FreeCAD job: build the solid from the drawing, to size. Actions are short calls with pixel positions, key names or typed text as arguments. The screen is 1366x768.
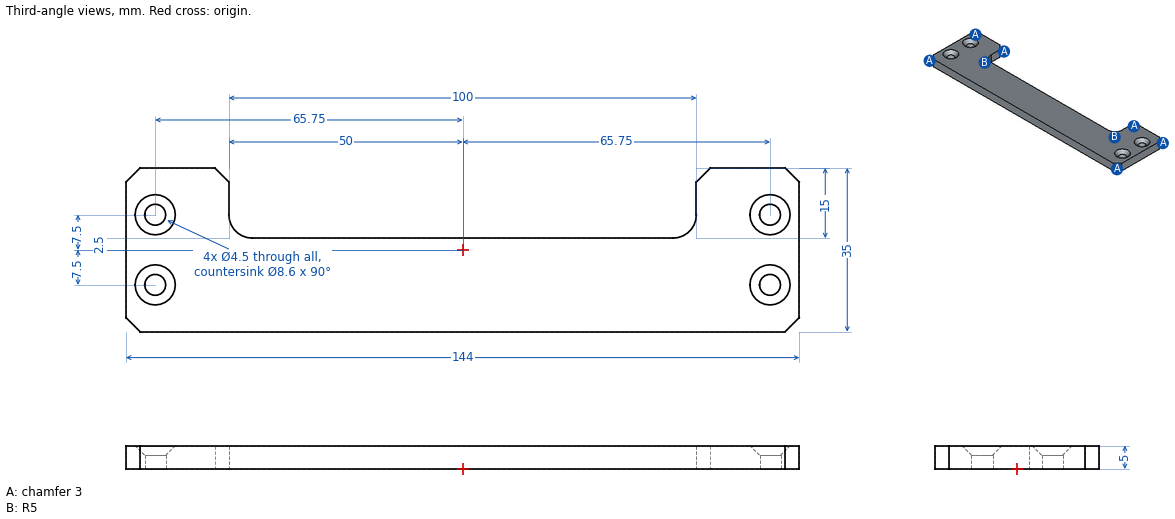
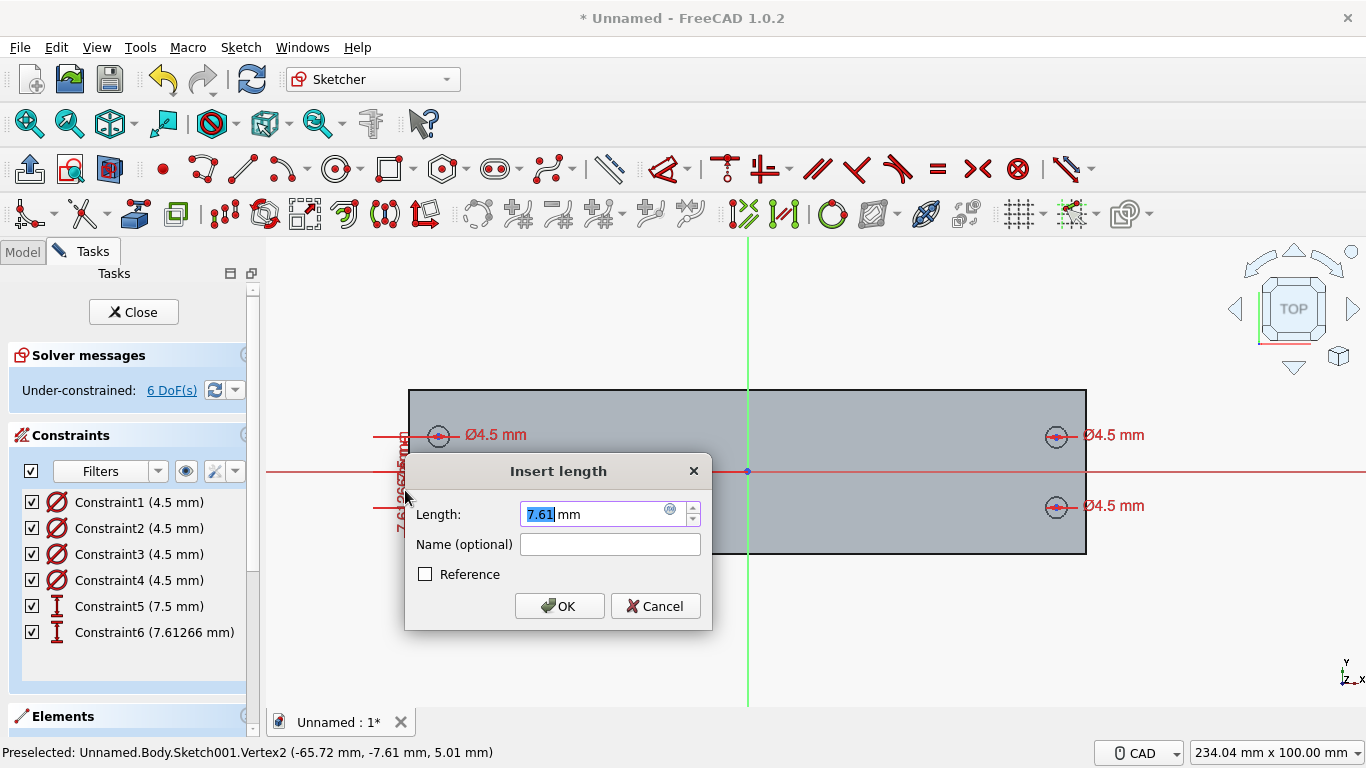
text(7.5)
key(Return)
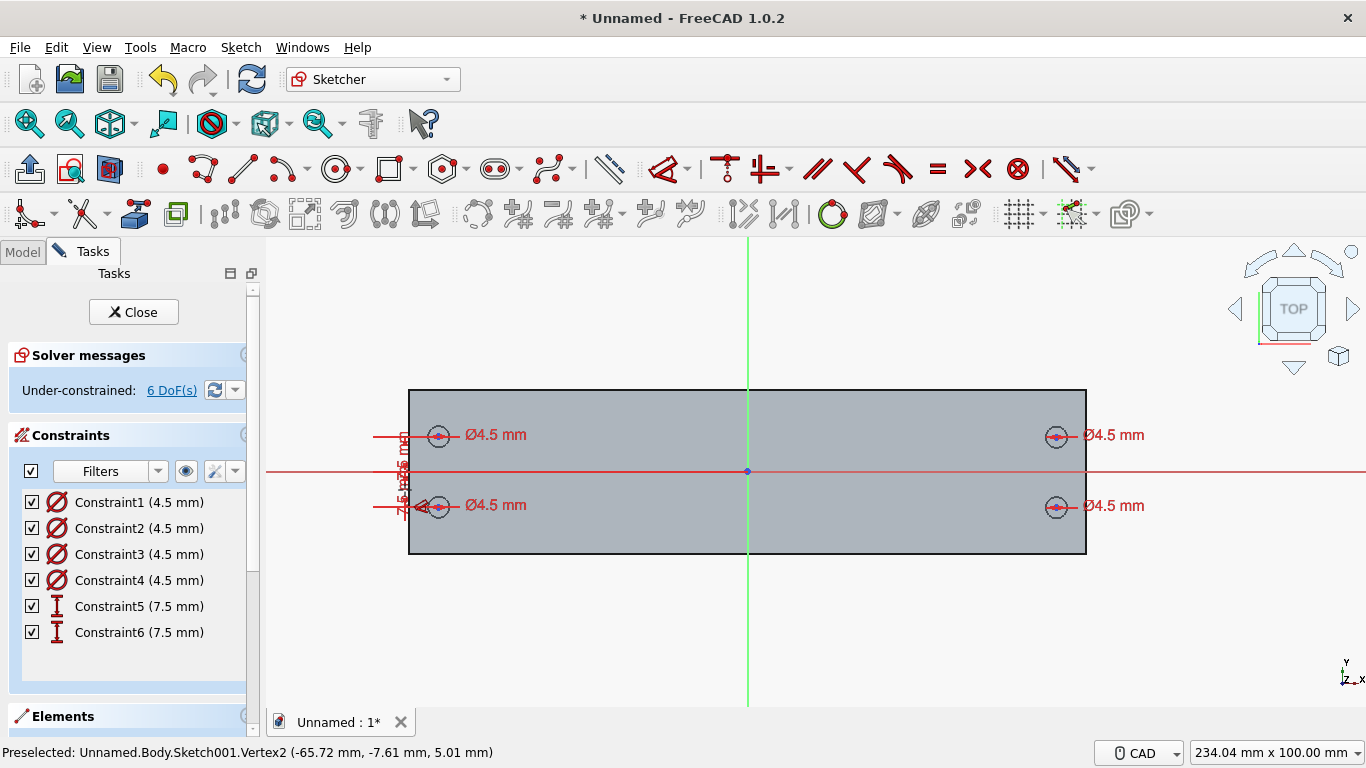
click(1056, 437)
click(1090, 455)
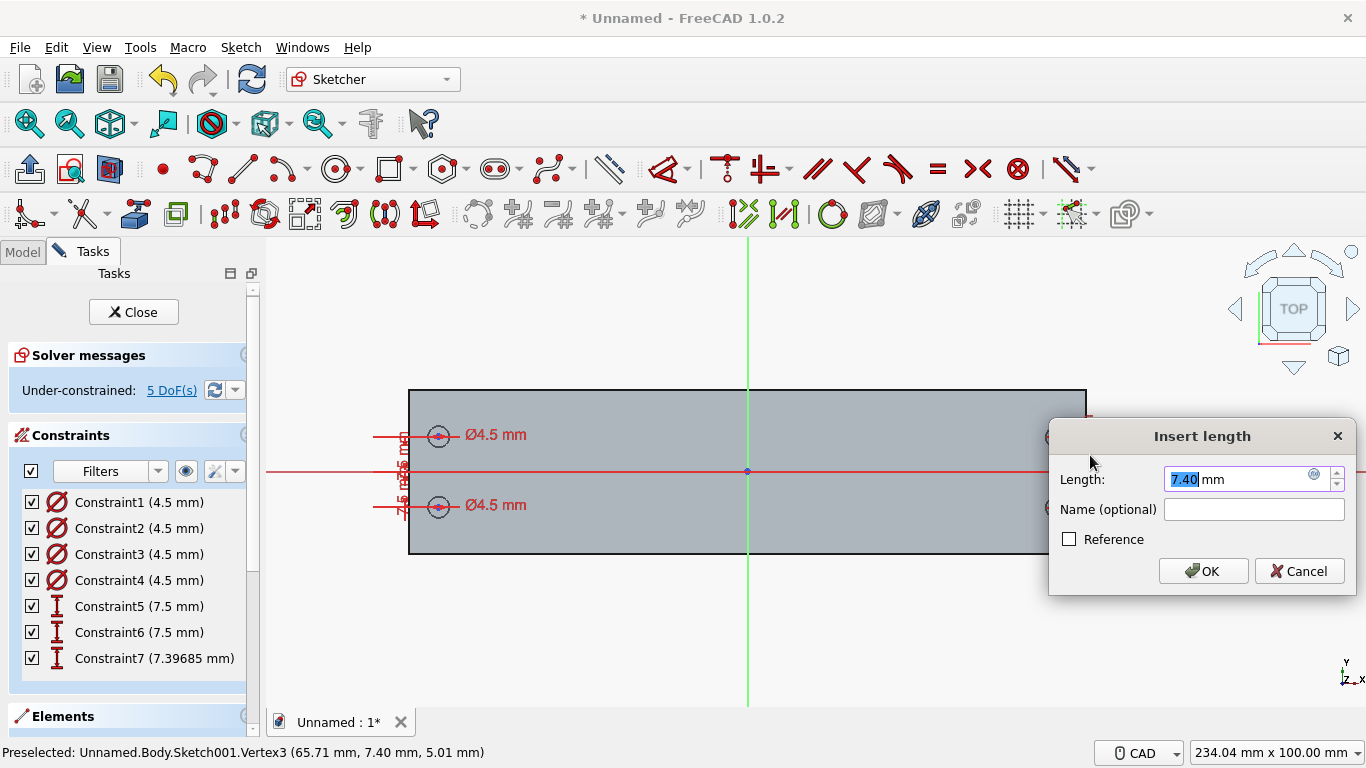
text(7.5)
key(Return)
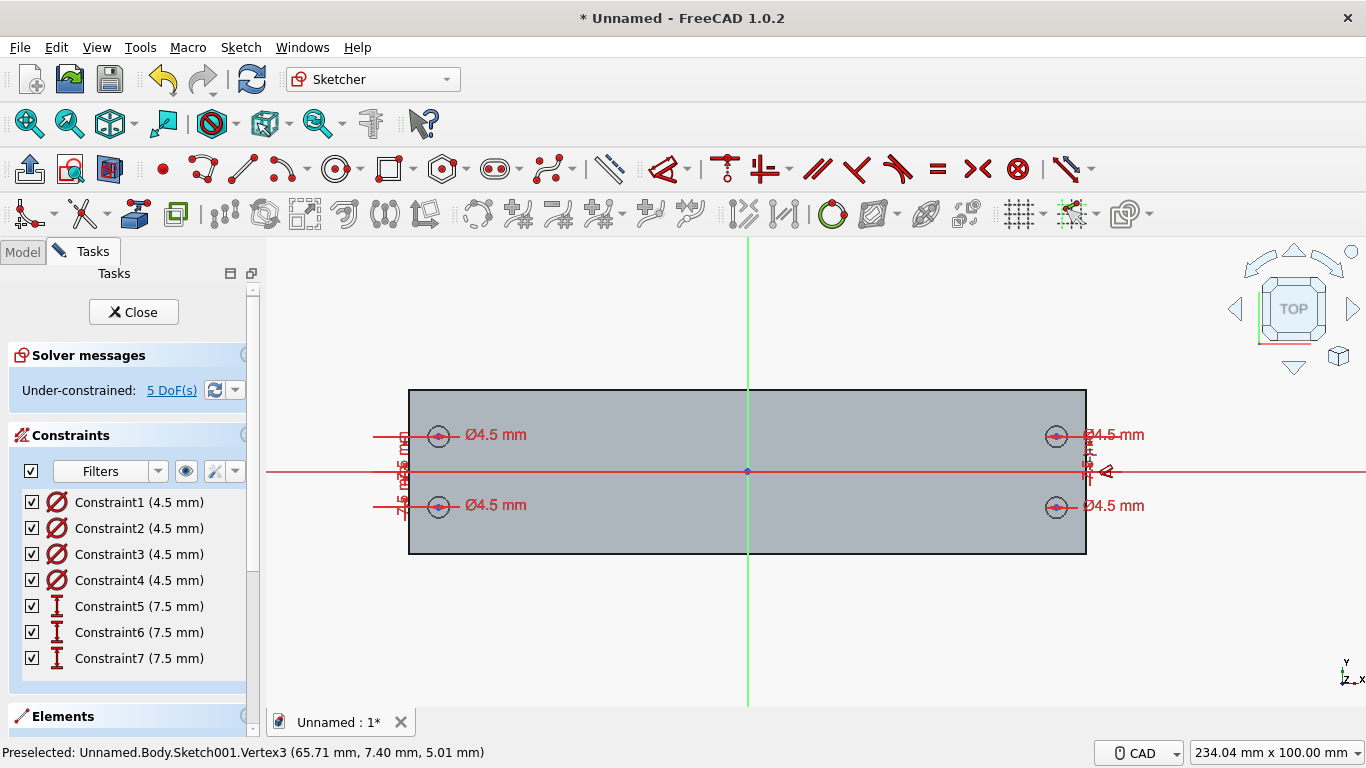
click(1056, 508)
click(1090, 490)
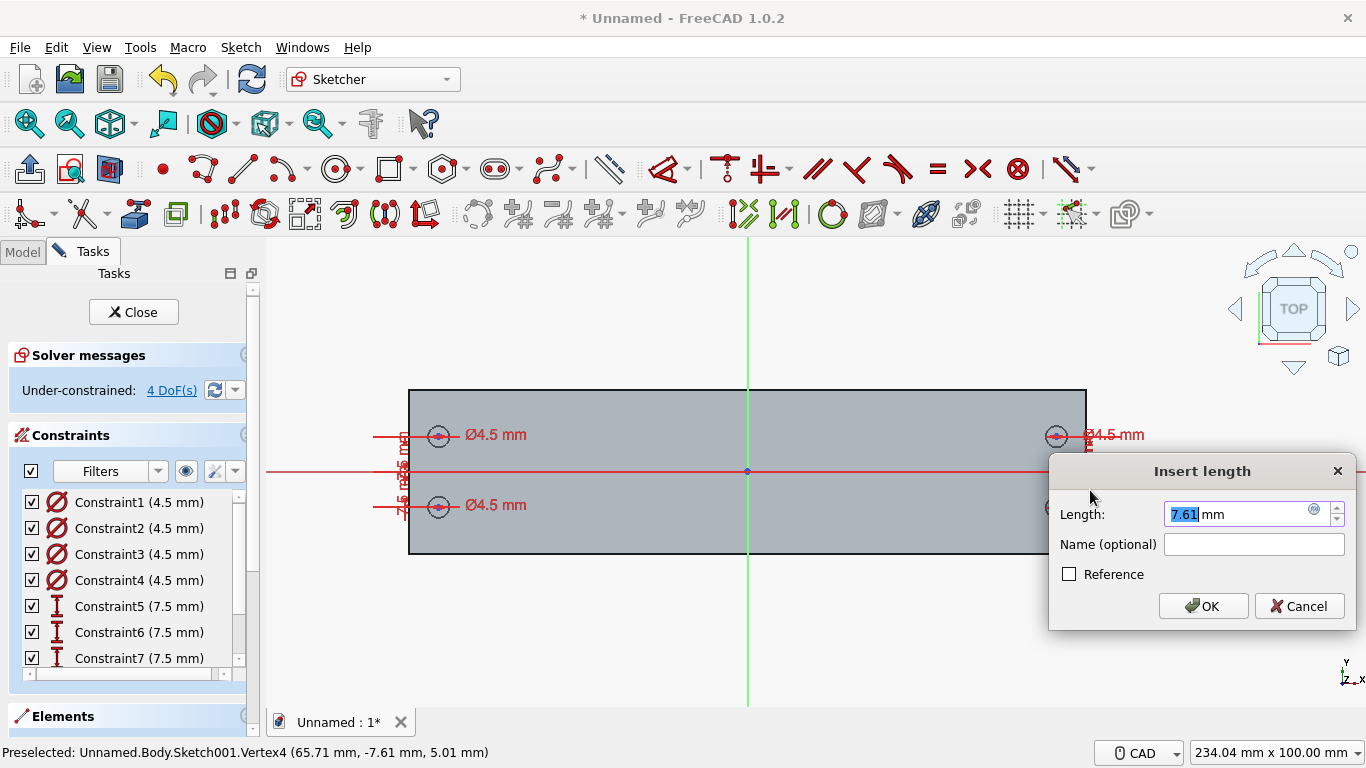
text(7.5)
key(Return)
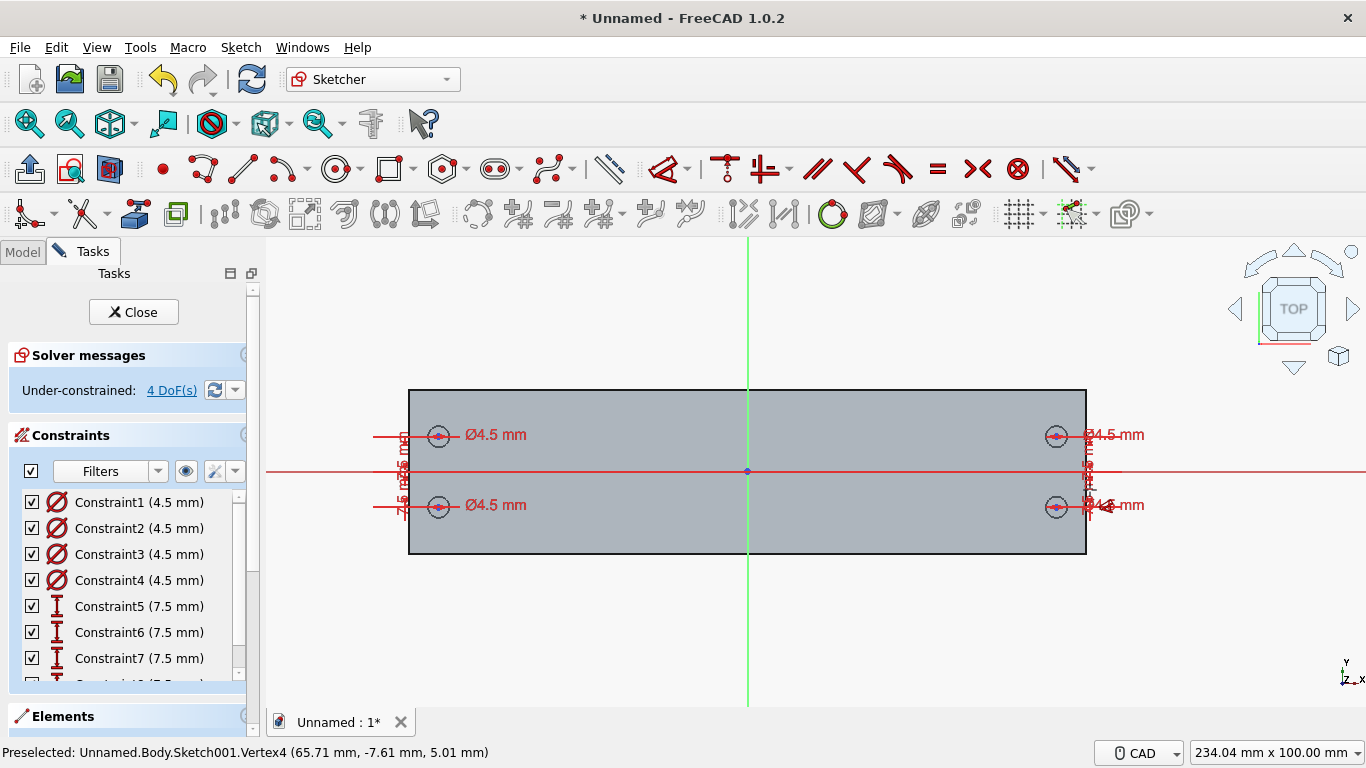
click(439, 437)
click(593, 403)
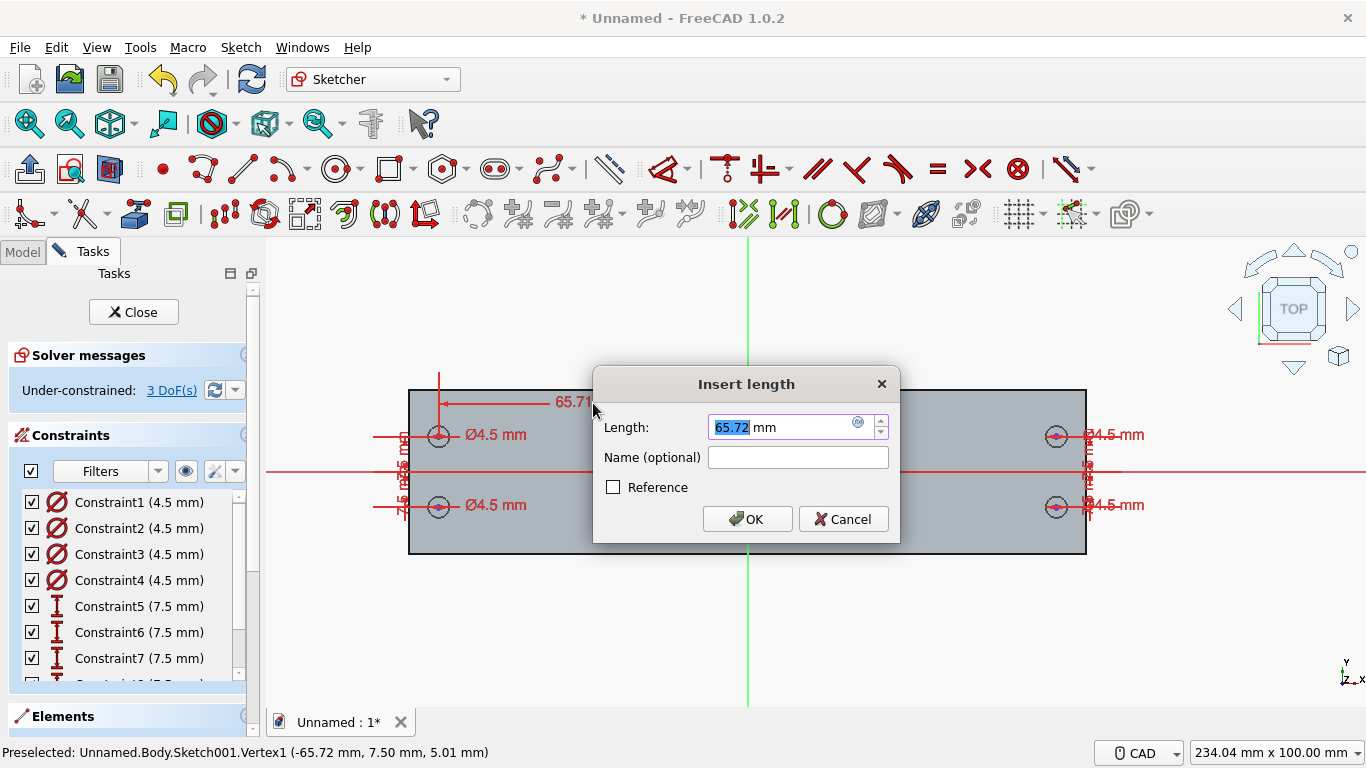
text(65.75)
key(Return)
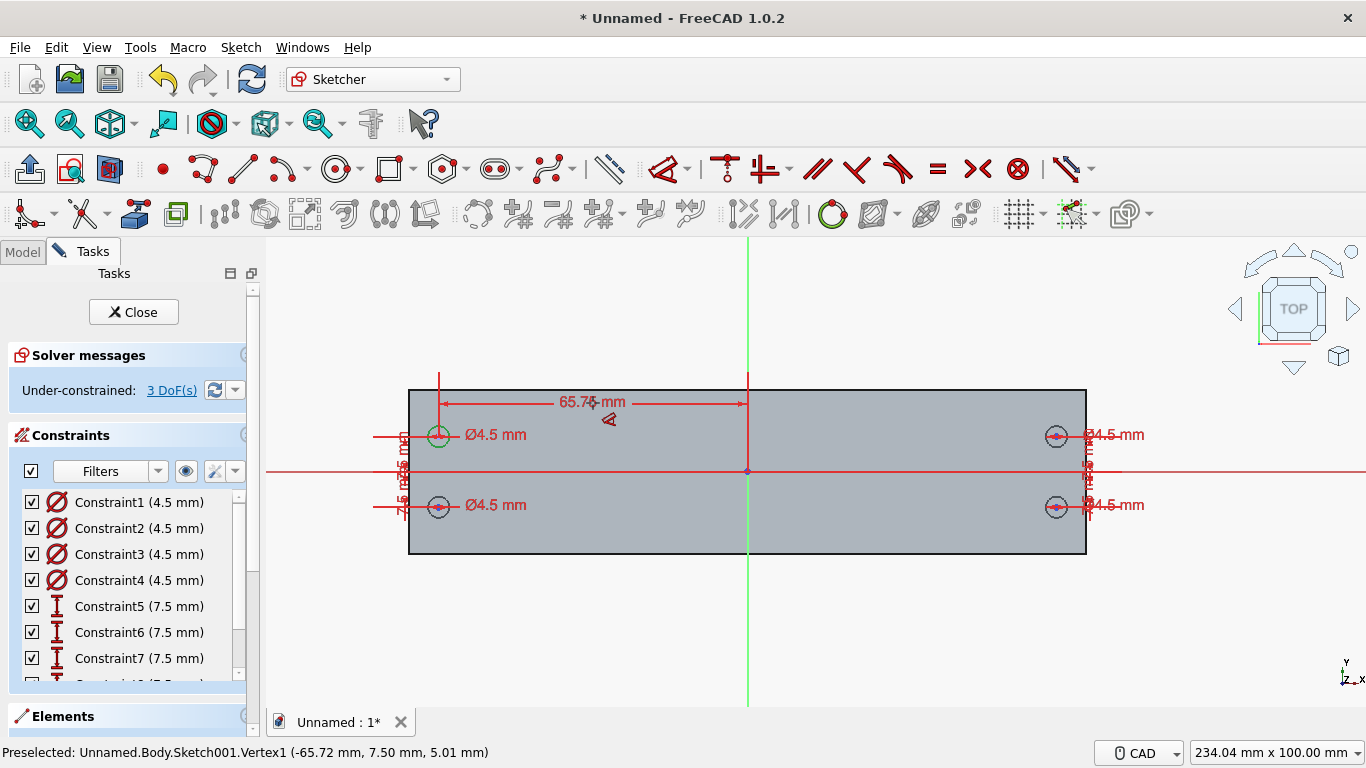
click(439, 507)
click(593, 541)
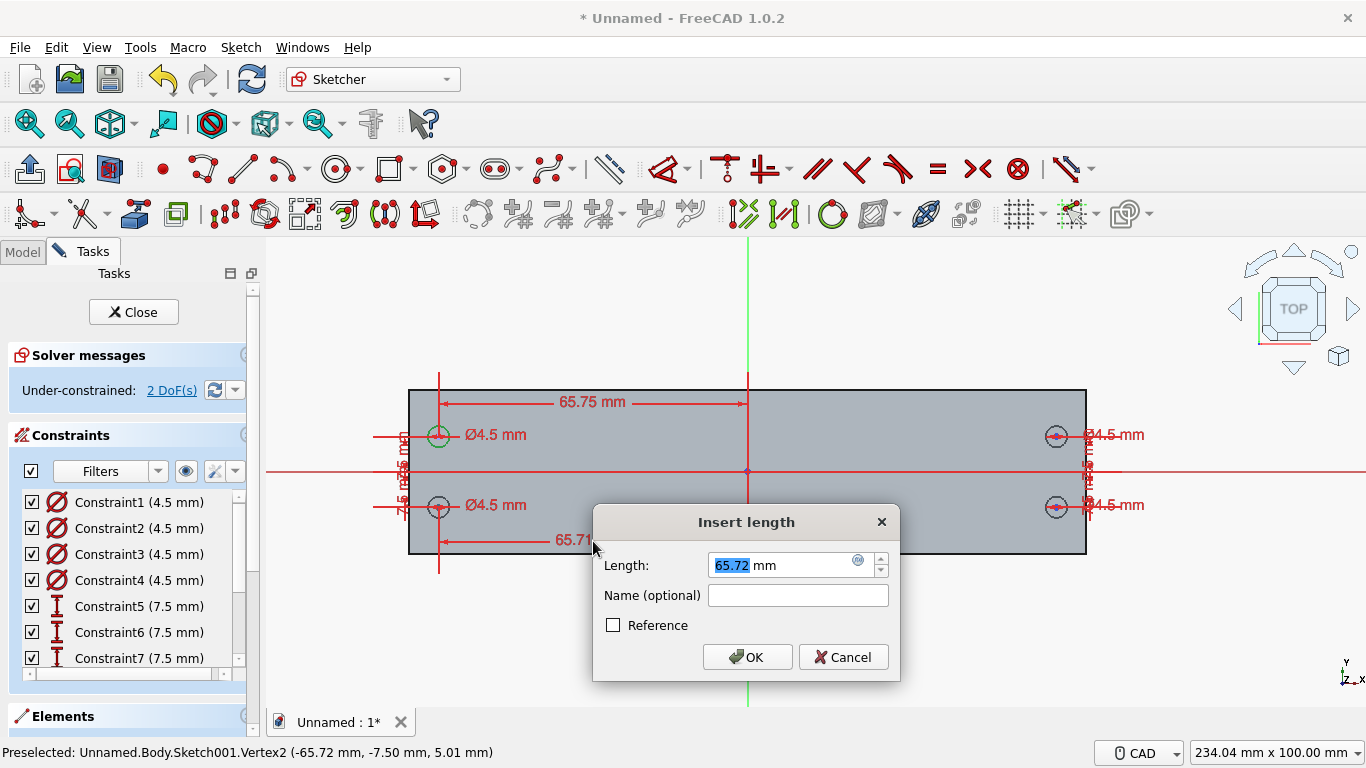
text(65.75)
key(Return)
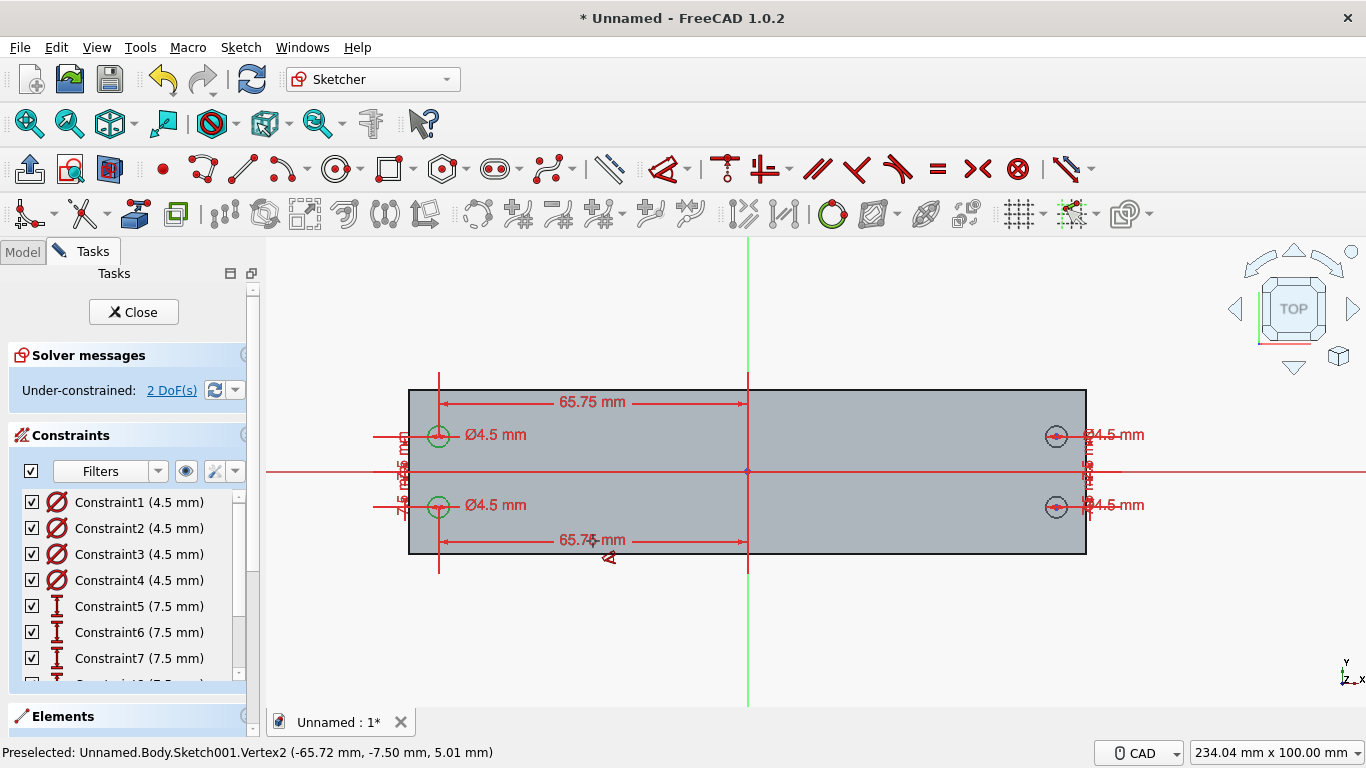
click(1056, 437)
click(902, 403)